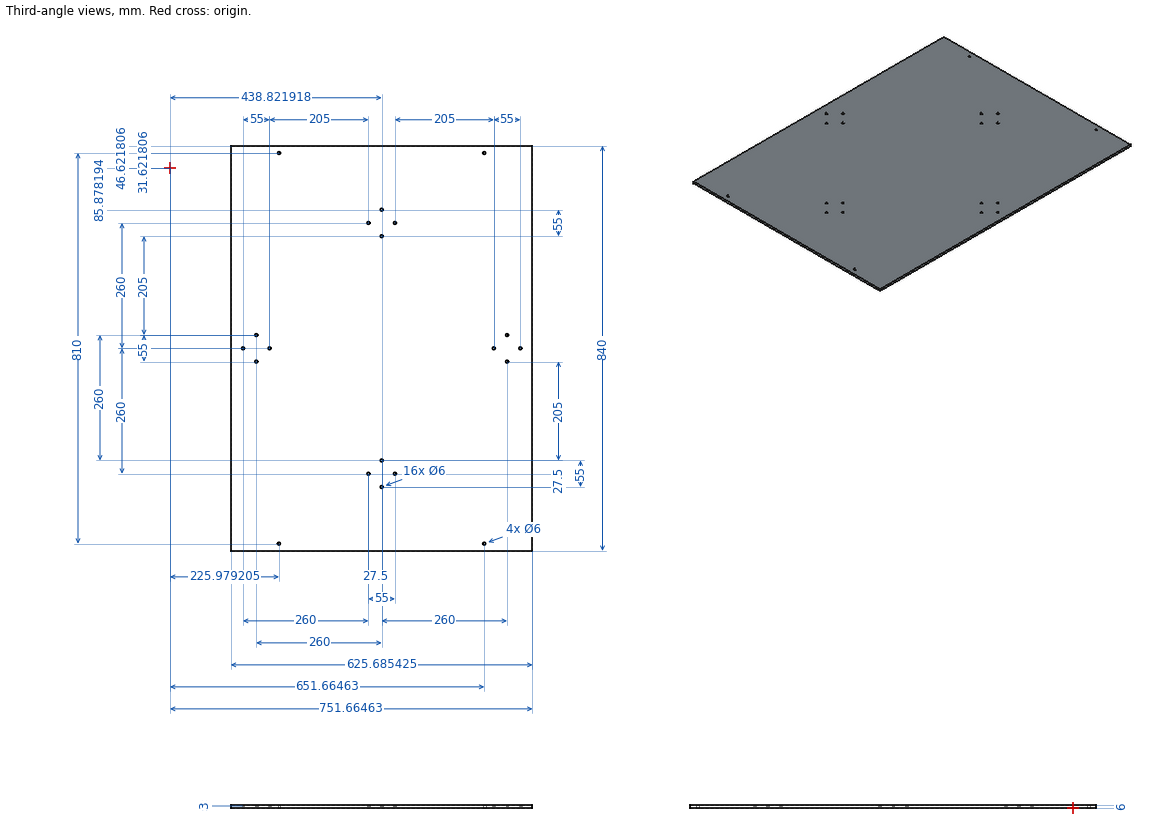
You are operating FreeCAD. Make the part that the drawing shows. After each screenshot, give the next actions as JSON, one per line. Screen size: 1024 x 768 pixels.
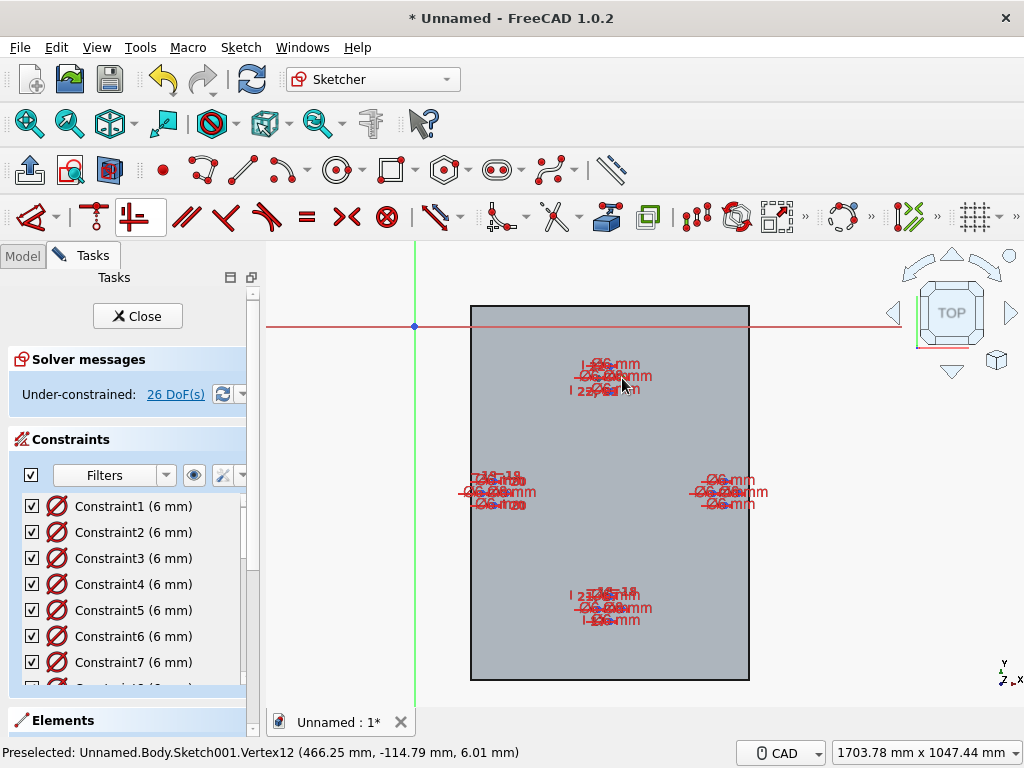
{"action": "key", "text": "h"}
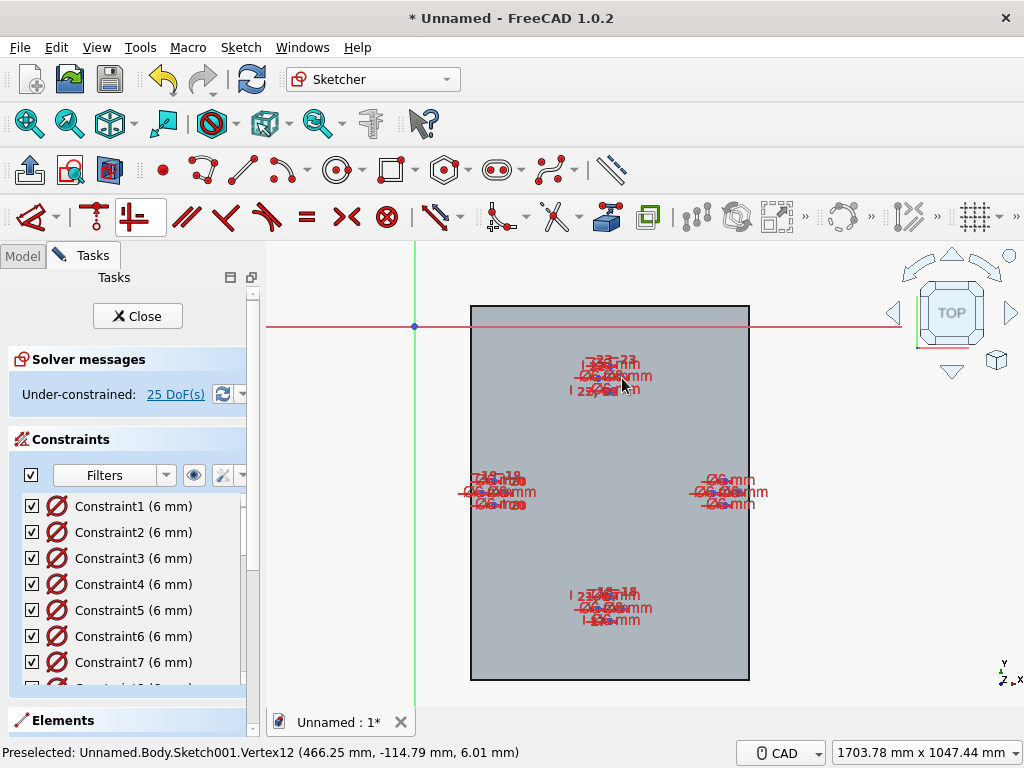
{"action": "left_click", "coordinate": [725, 506]}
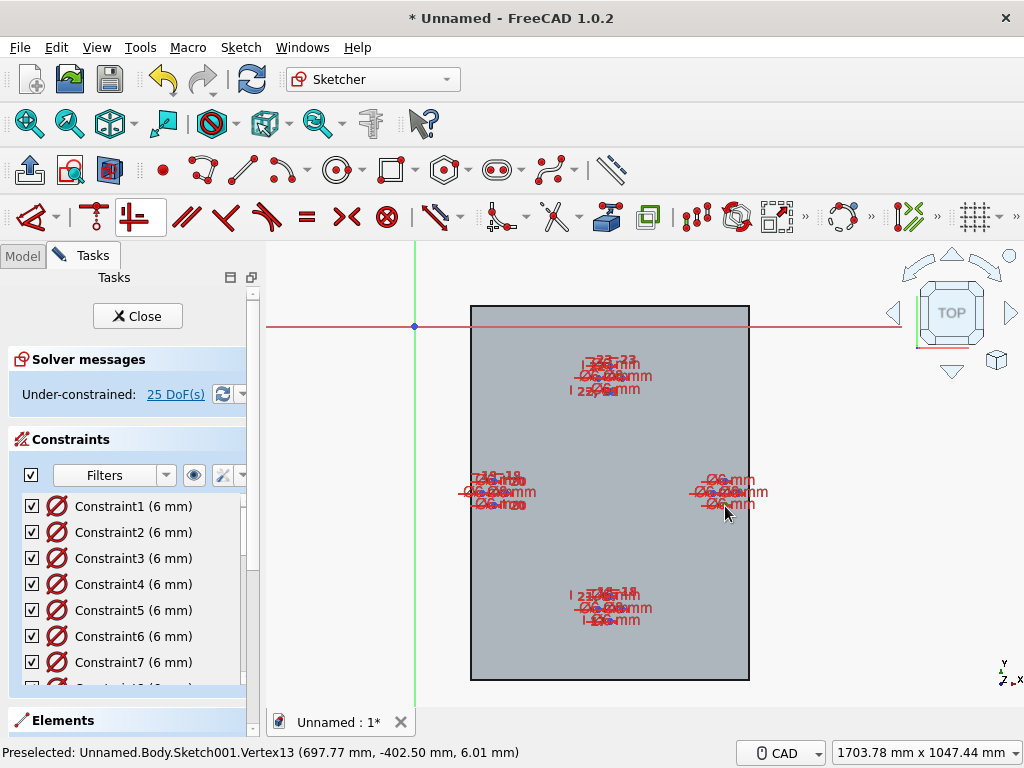
{"action": "left_click", "coordinate": [725, 482]}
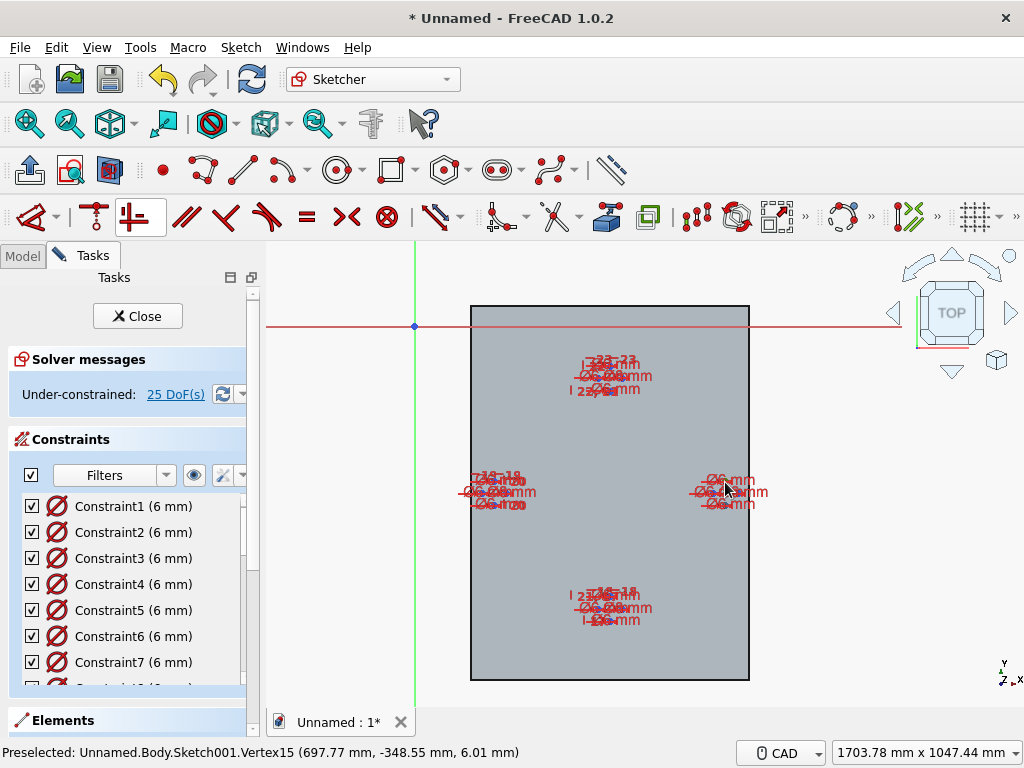
{"action": "left_click", "coordinate": [160, 218]}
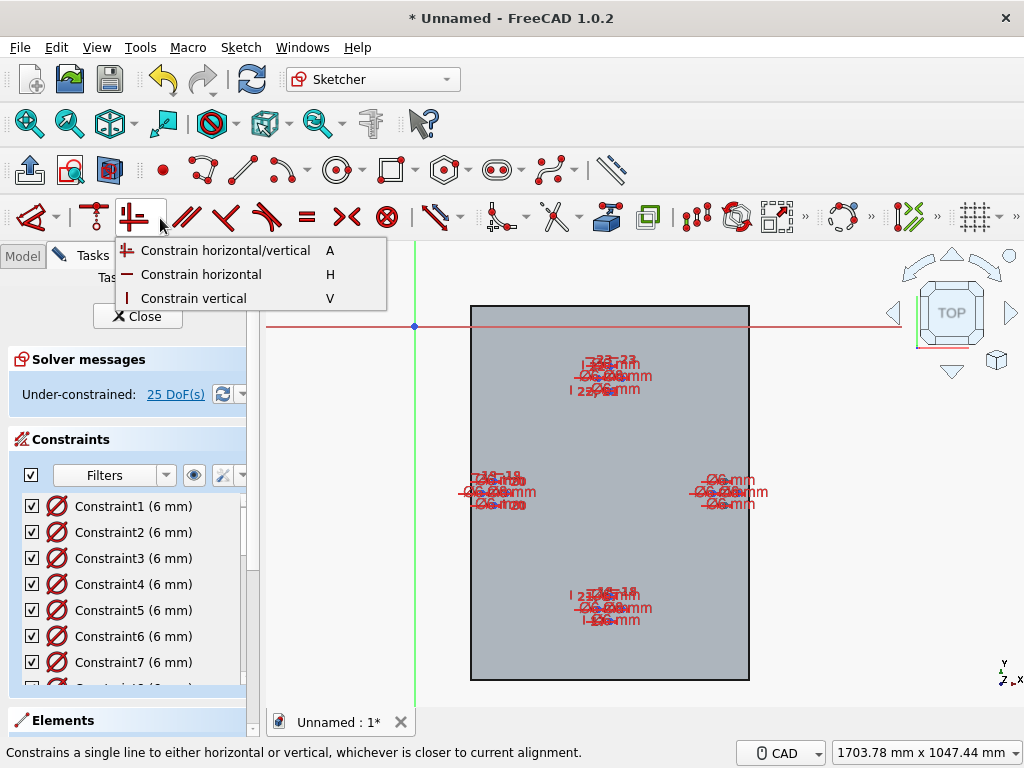
{"action": "left_click", "coordinate": [251, 298]}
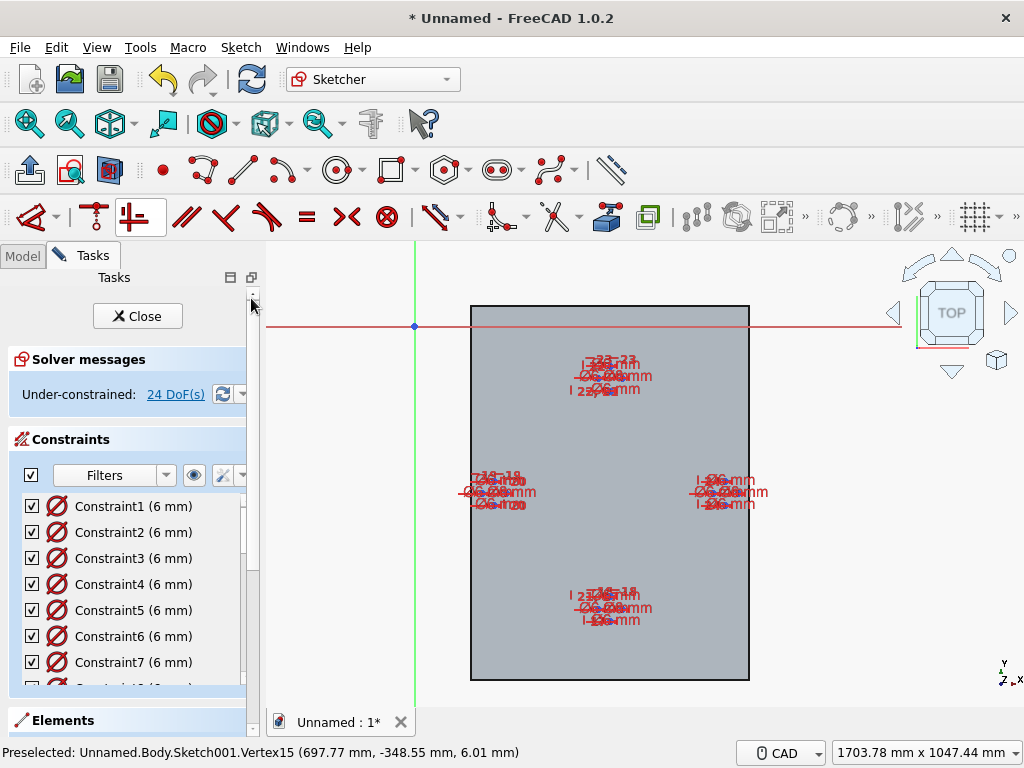
{"action": "left_click", "coordinate": [713, 494]}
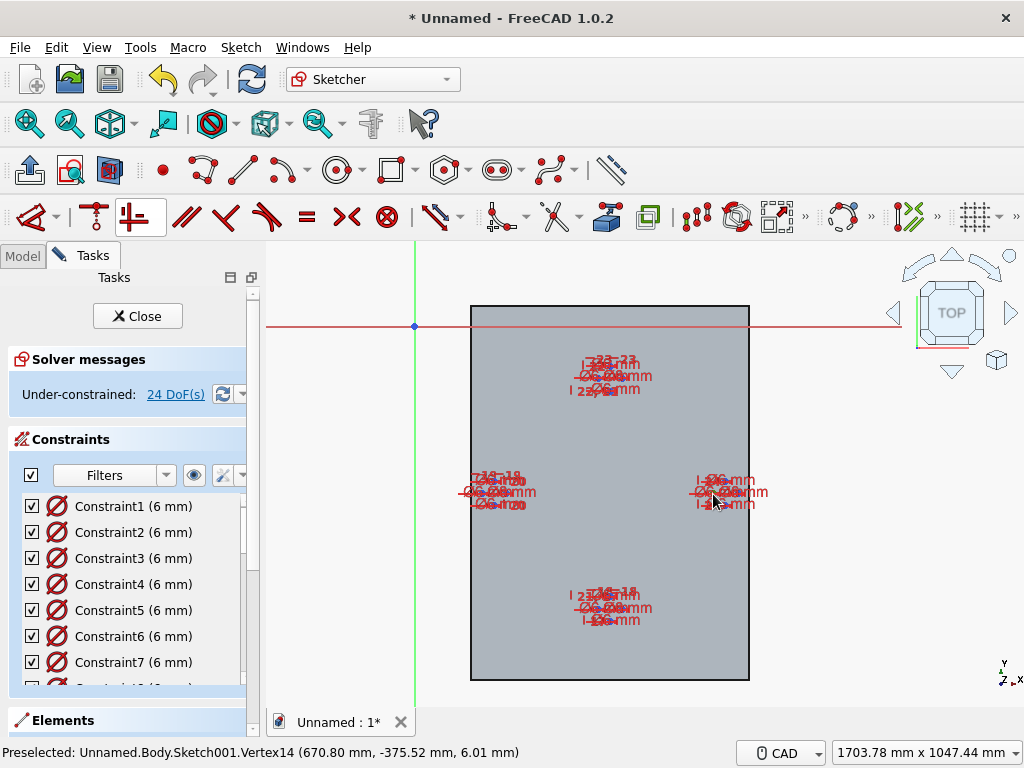
{"action": "left_click", "coordinate": [738, 494]}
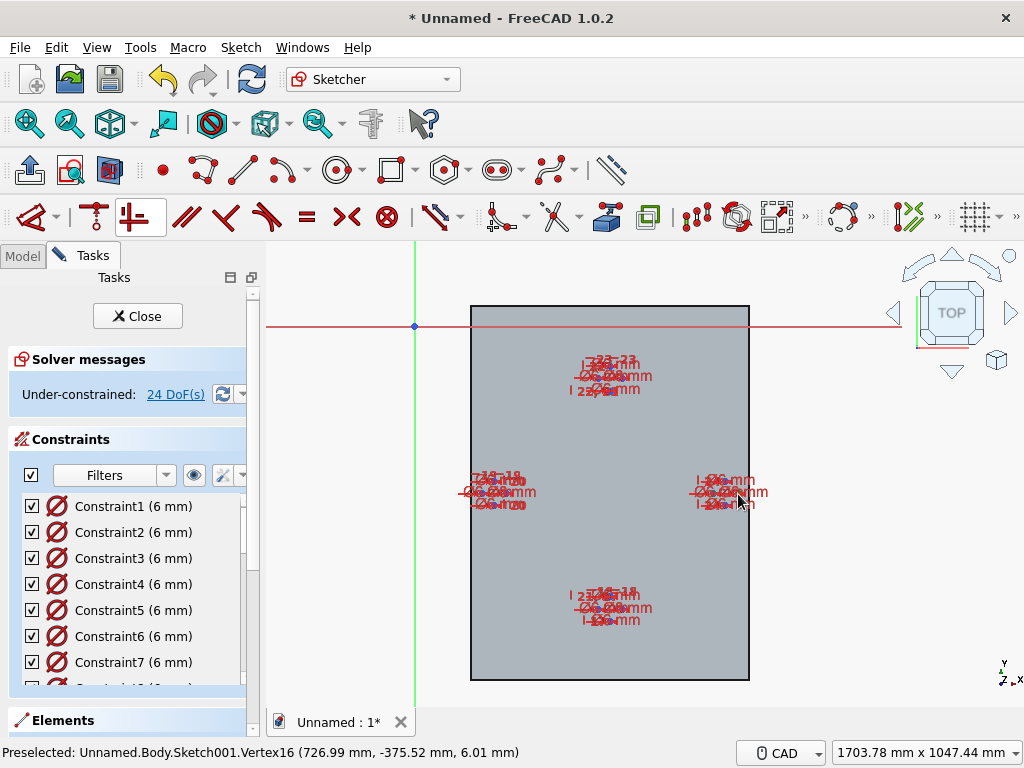
{"action": "left_click", "coordinate": [160, 218]}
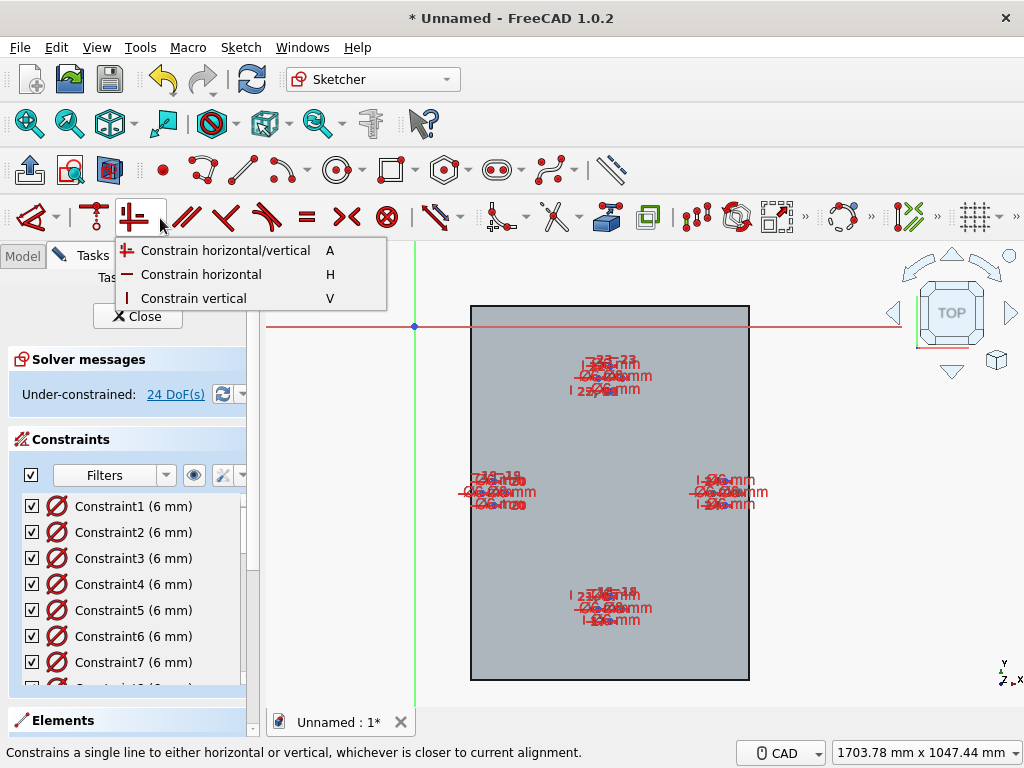
{"action": "left_click", "coordinate": [251, 274]}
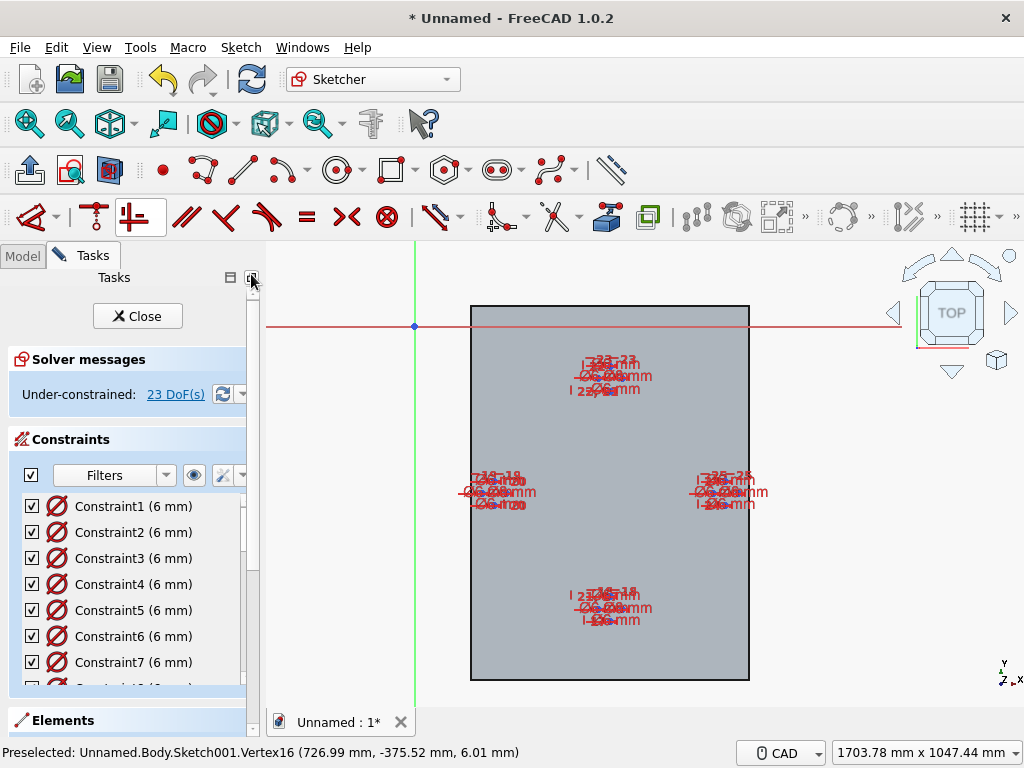
{"action": "left_click", "coordinate": [32, 218]}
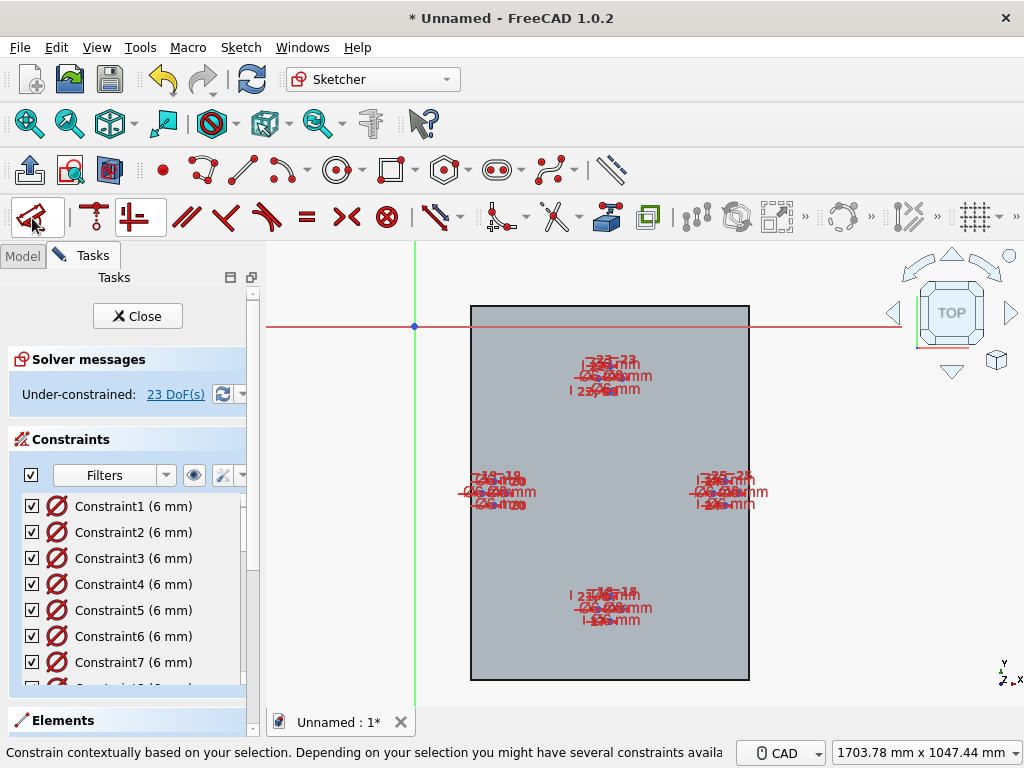
{"action": "scroll", "coordinate": [610, 622], "scroll_direction": "up", "scroll_amount": 3}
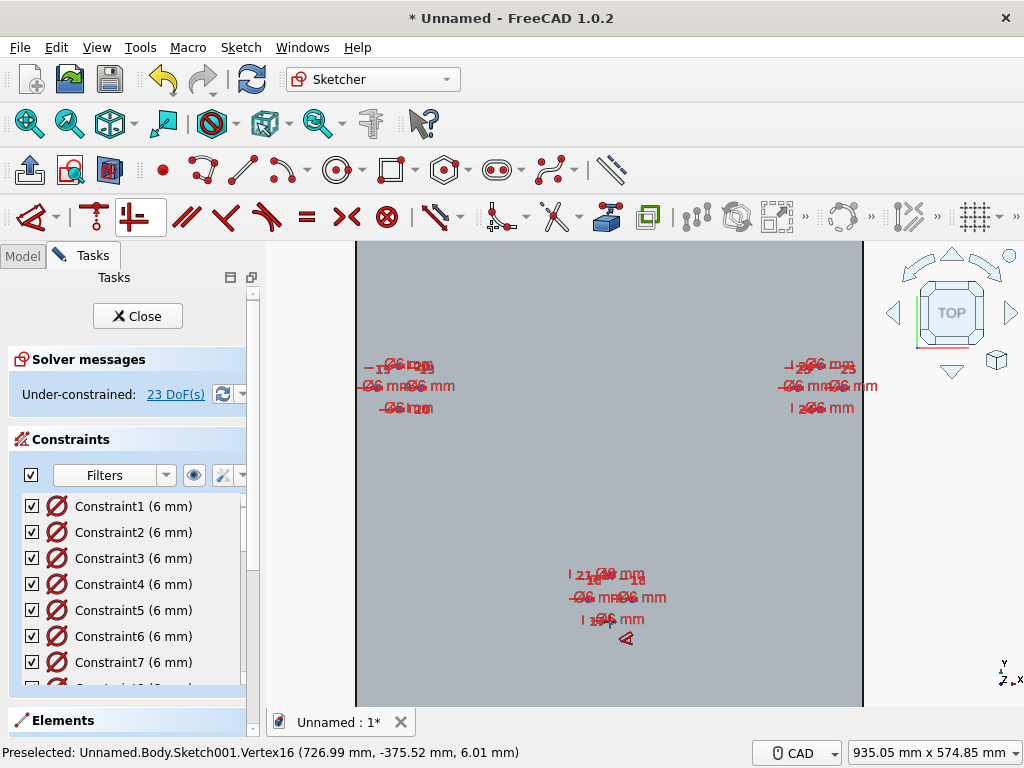
{"action": "left_click", "coordinate": [610, 621]}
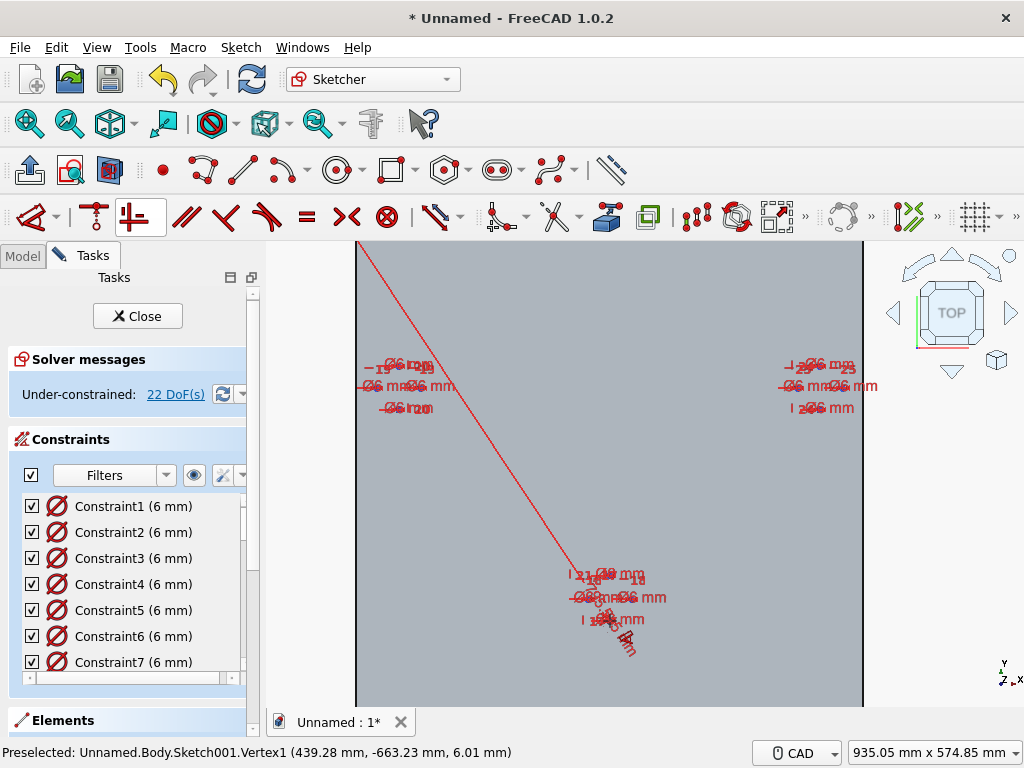
{"action": "left_click", "coordinate": [610, 576]}
{"action": "left_click", "coordinate": [644, 588]}